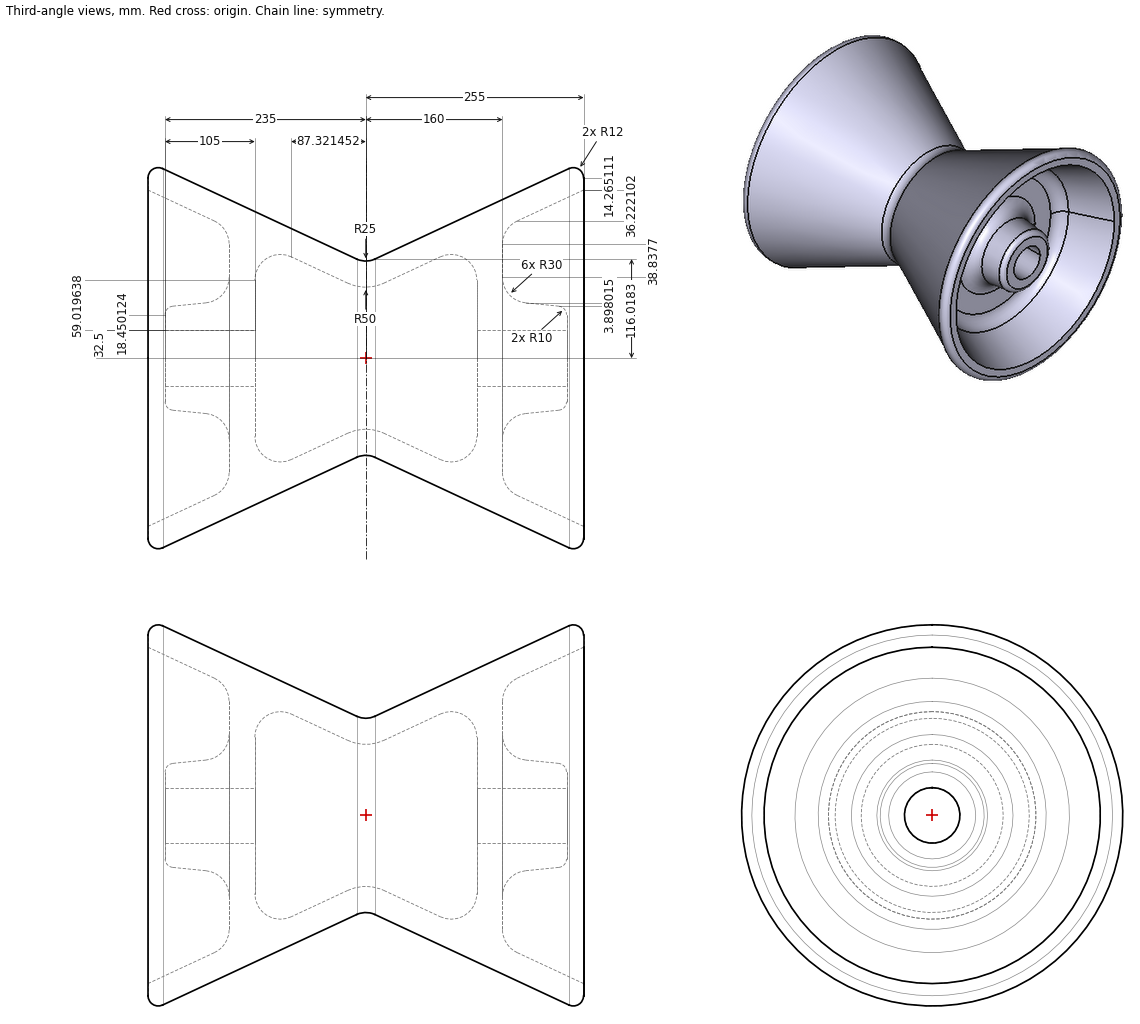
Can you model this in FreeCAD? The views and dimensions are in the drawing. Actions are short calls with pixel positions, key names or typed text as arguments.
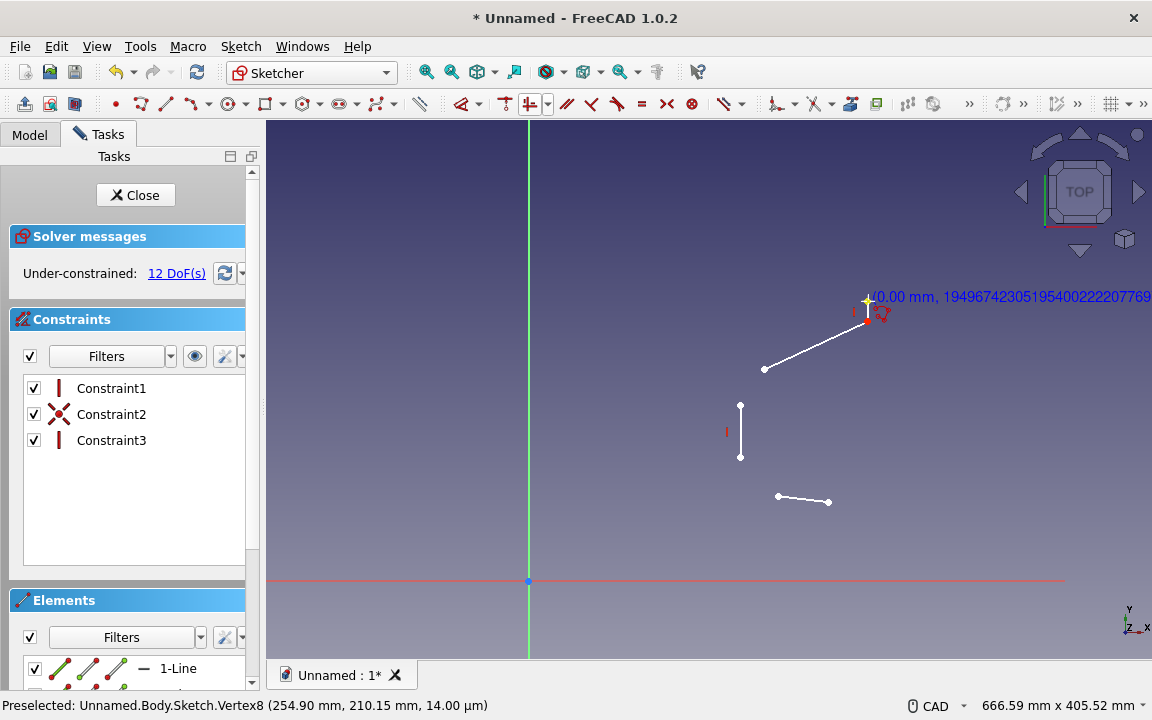
click(166, 104)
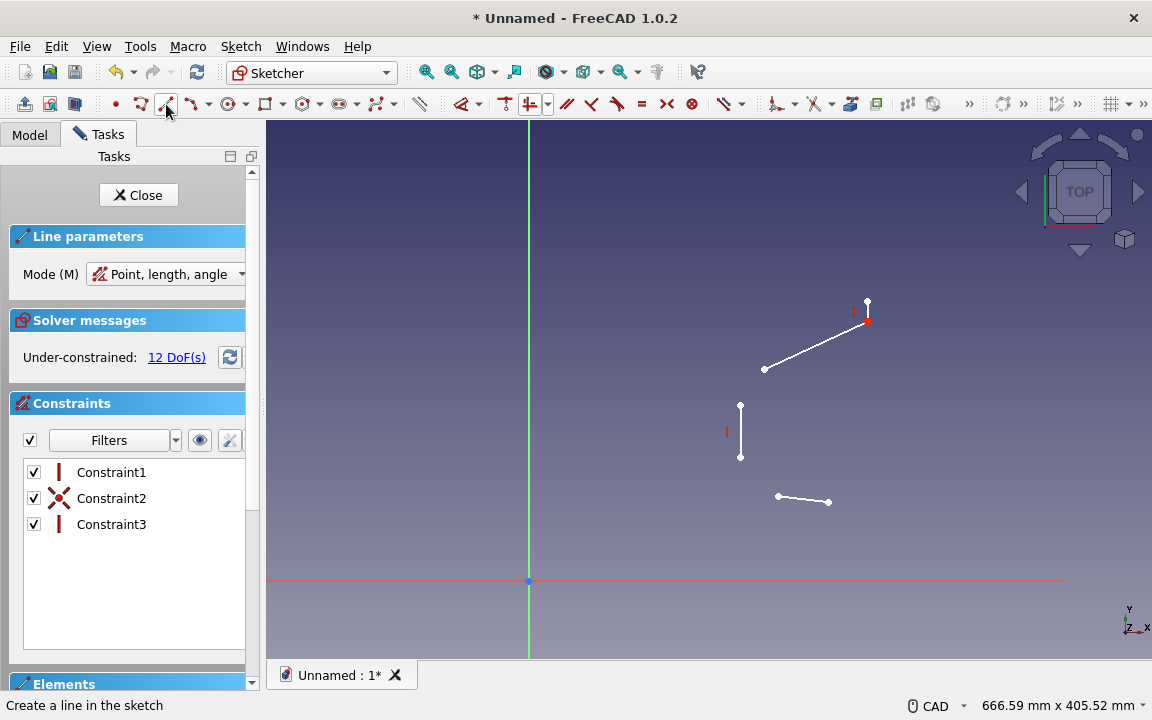
click(845, 286)
click(543, 427)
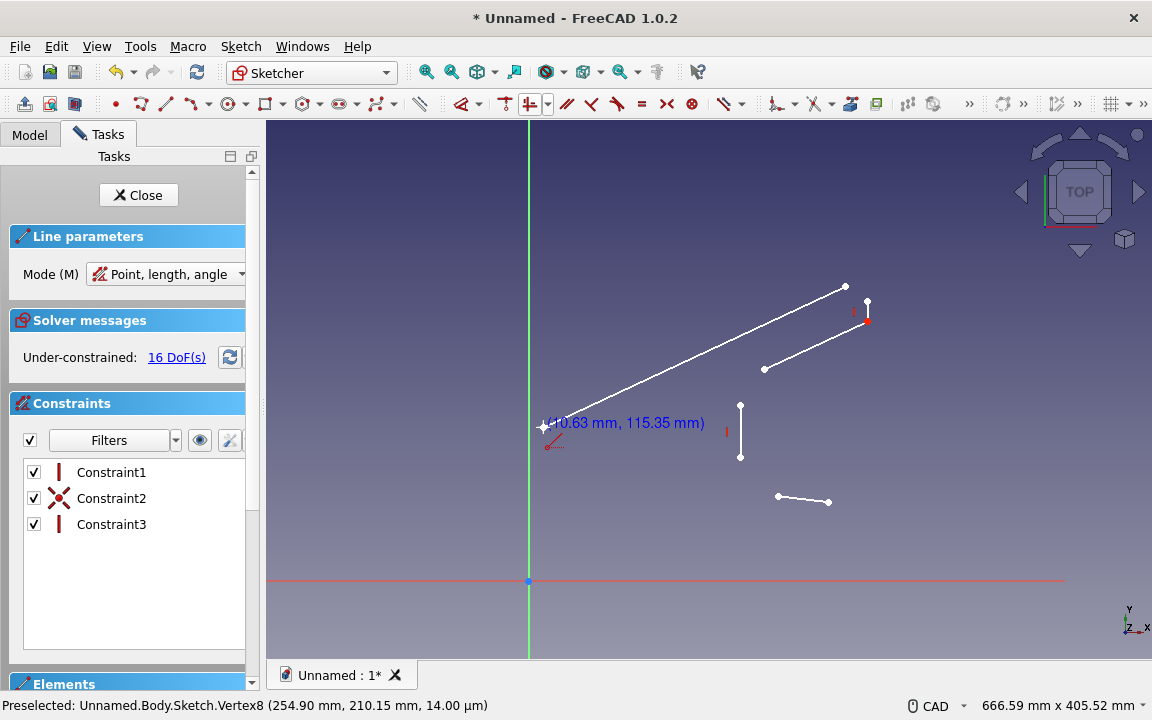
click(515, 427)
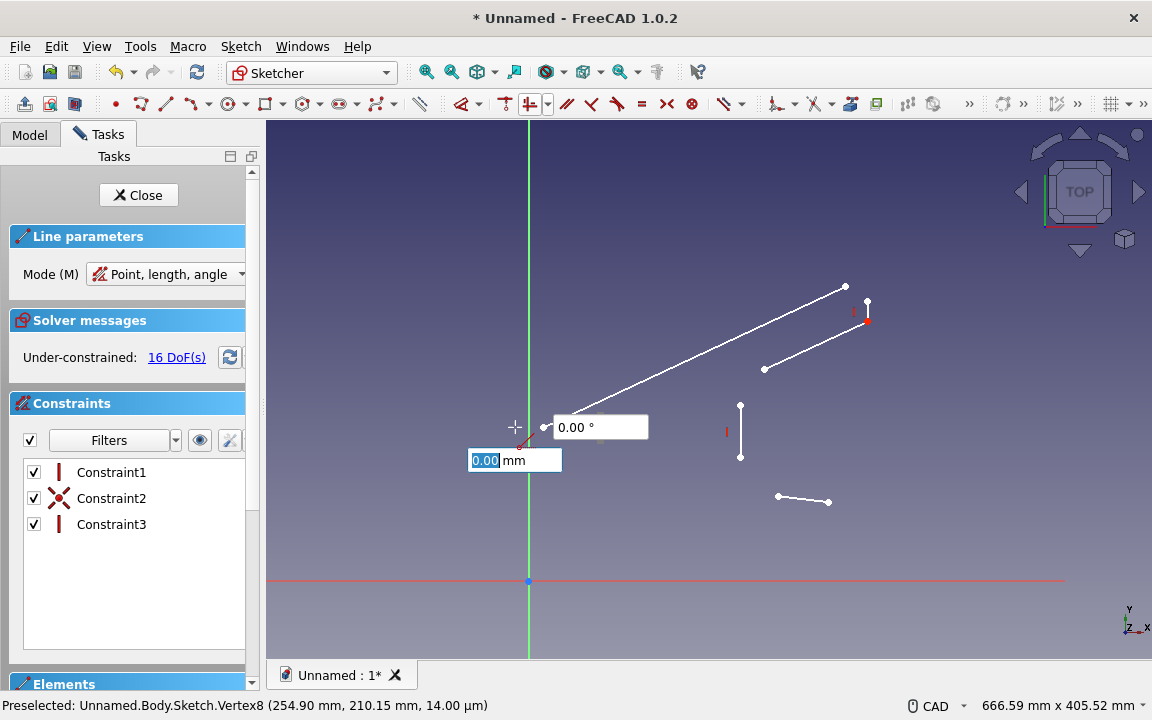
scroll(867, 300, down, 2)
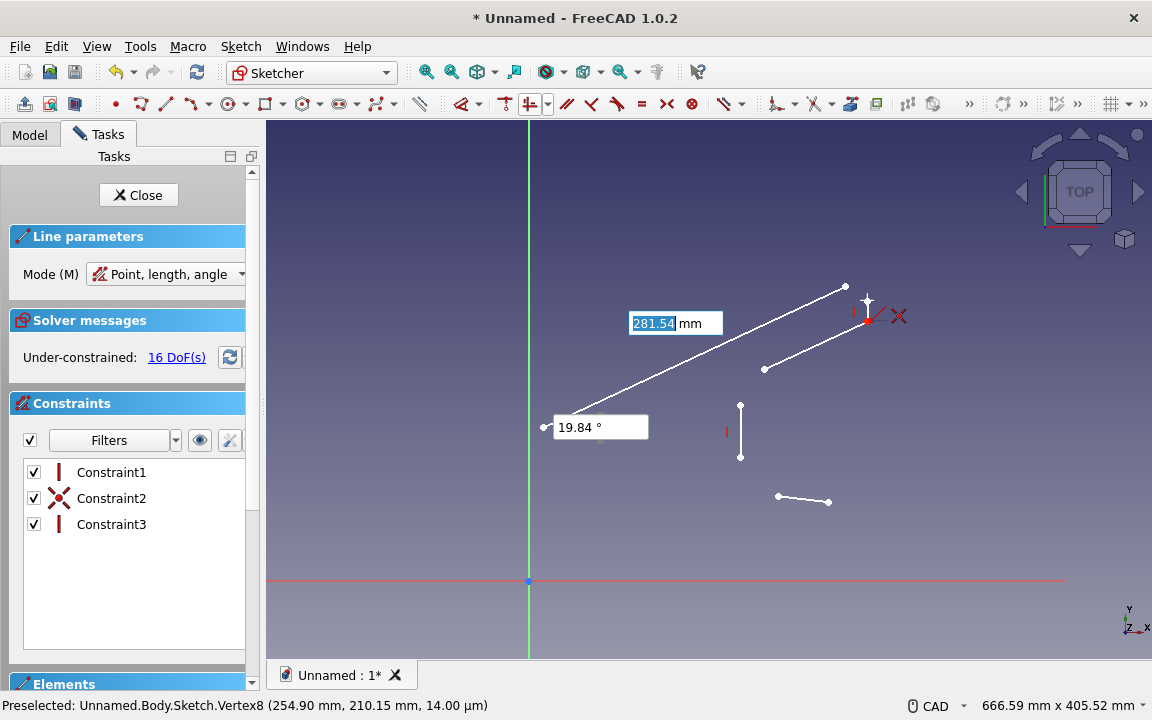
click(429, 291)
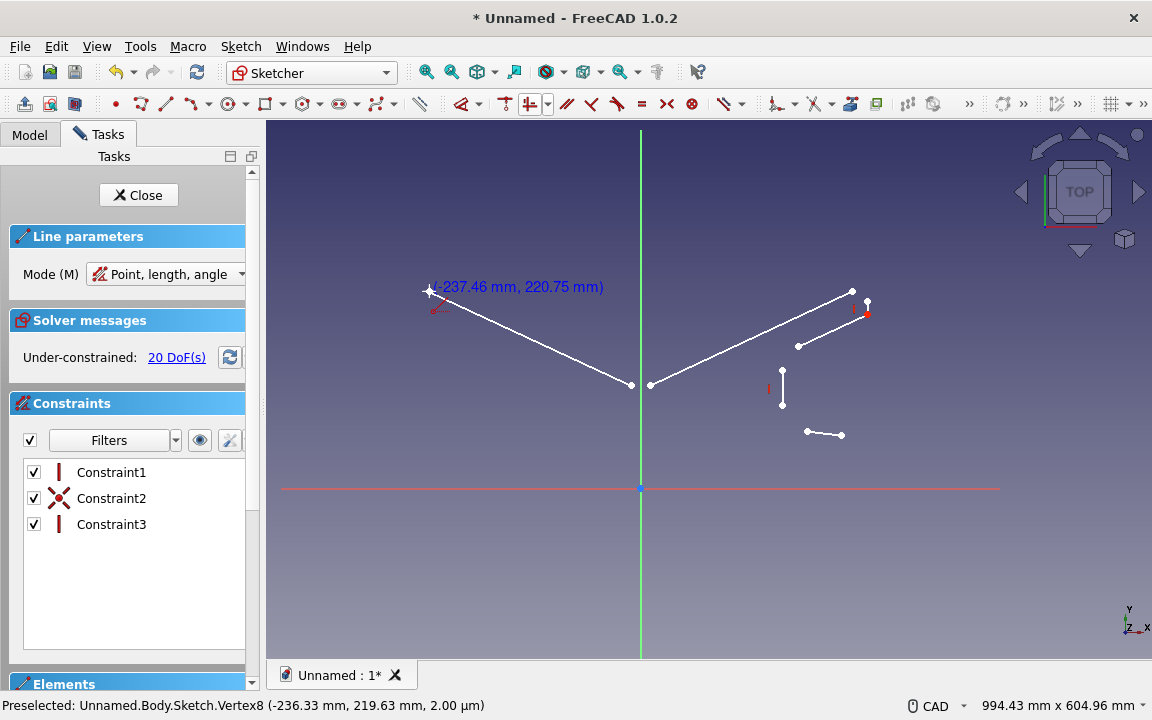
key(g)
key(m)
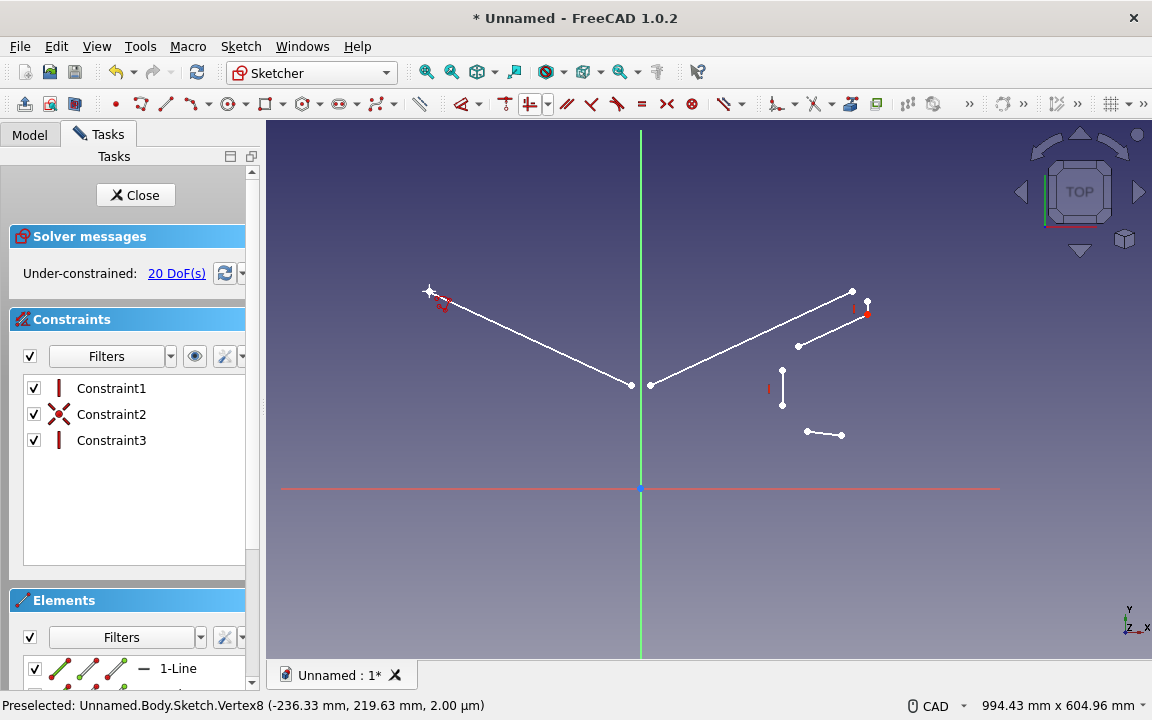
click(413, 301)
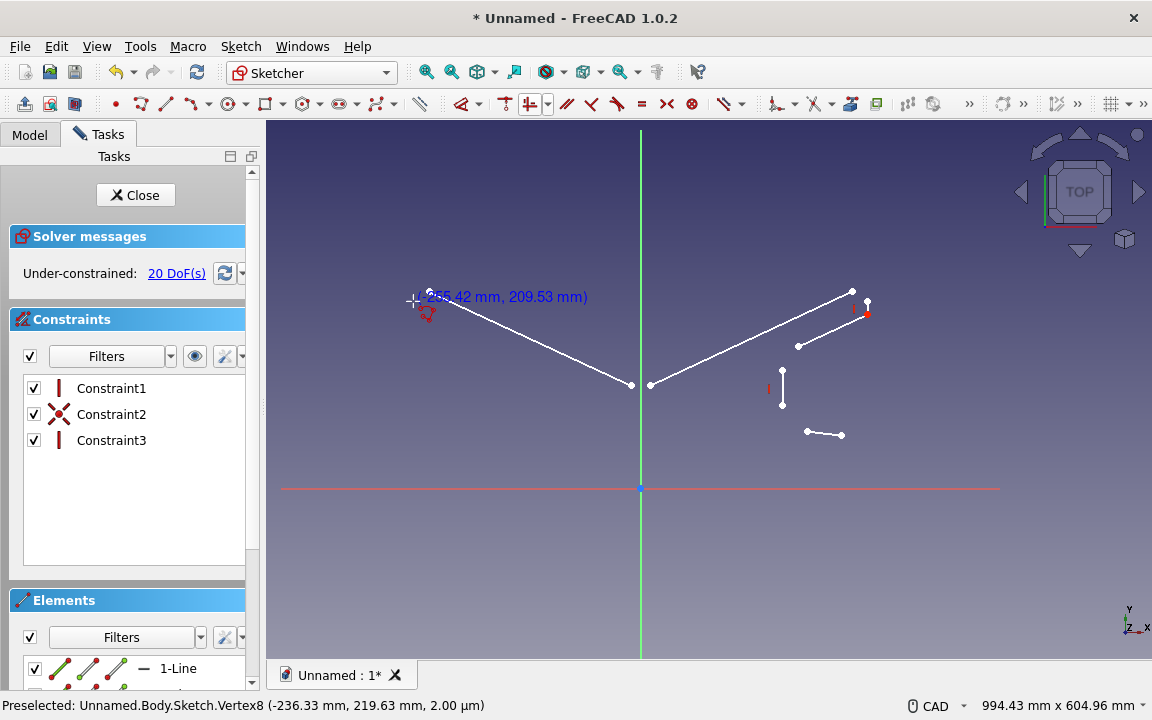
scroll(413, 313, up, 2)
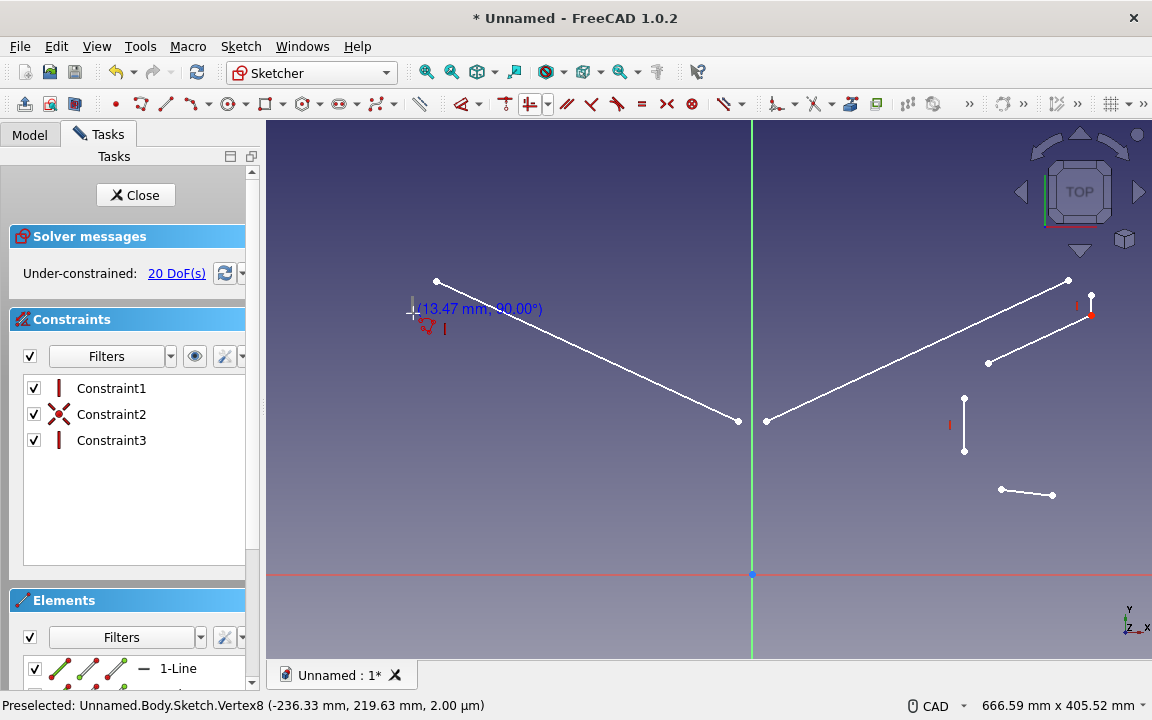
click(413, 313)
click(517, 361)
right_click(517, 361)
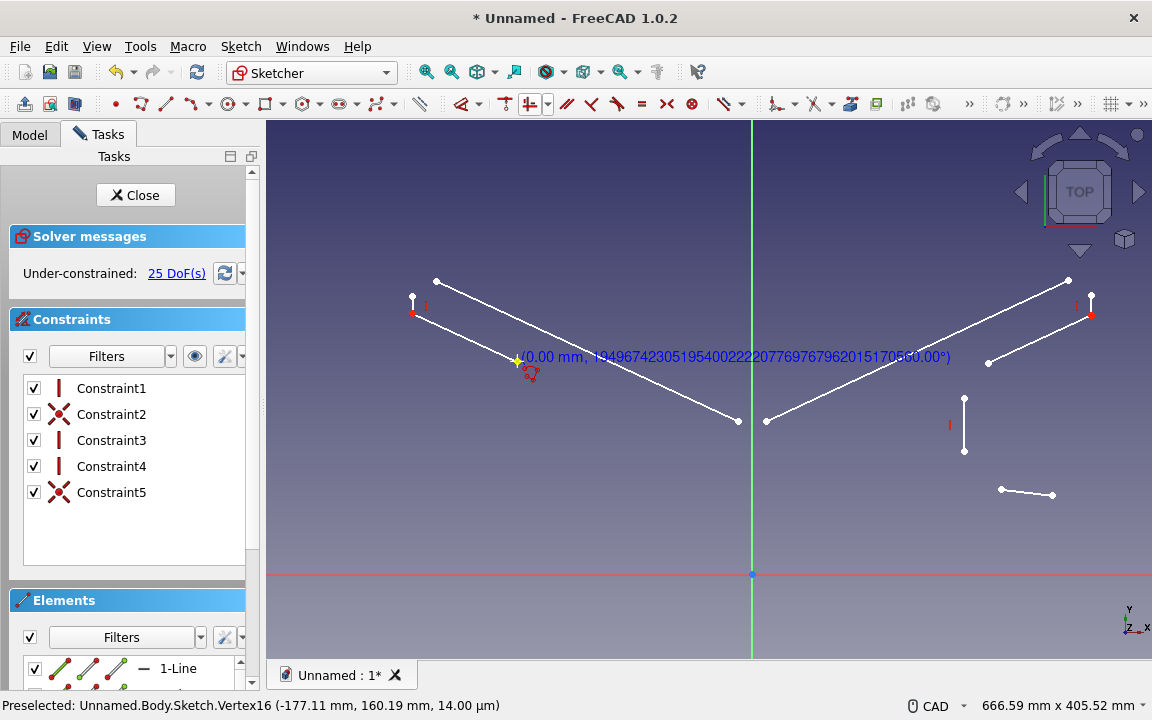
click(166, 104)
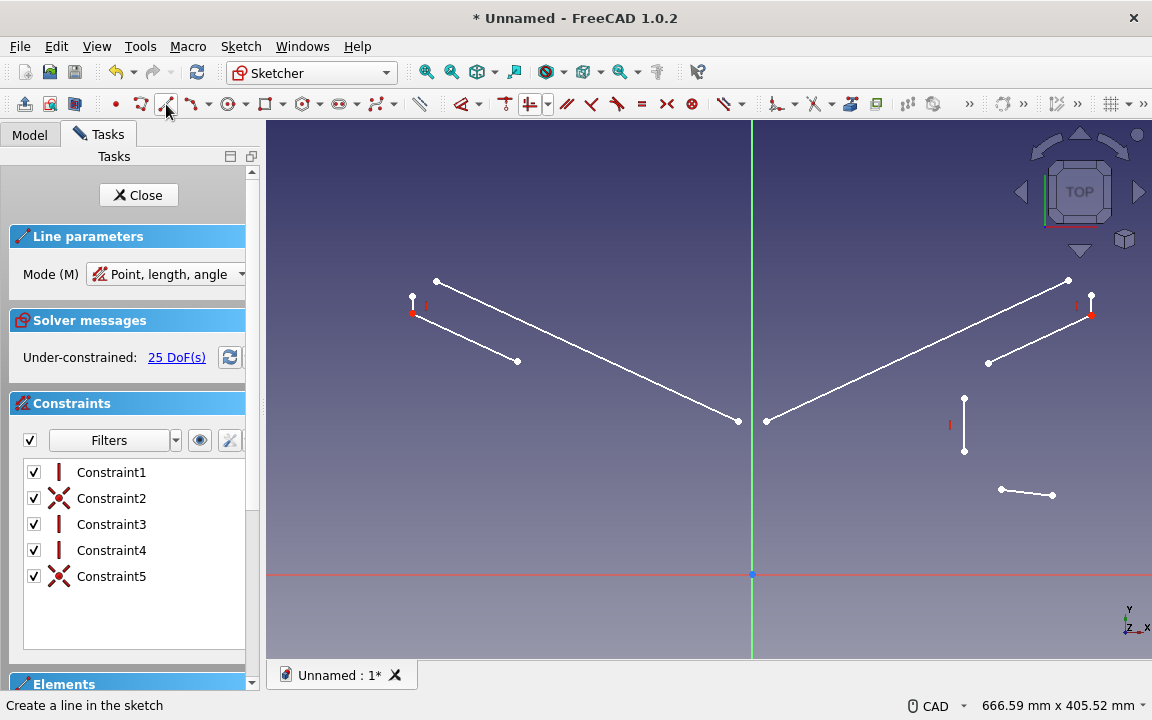
click(540, 397)
click(540, 449)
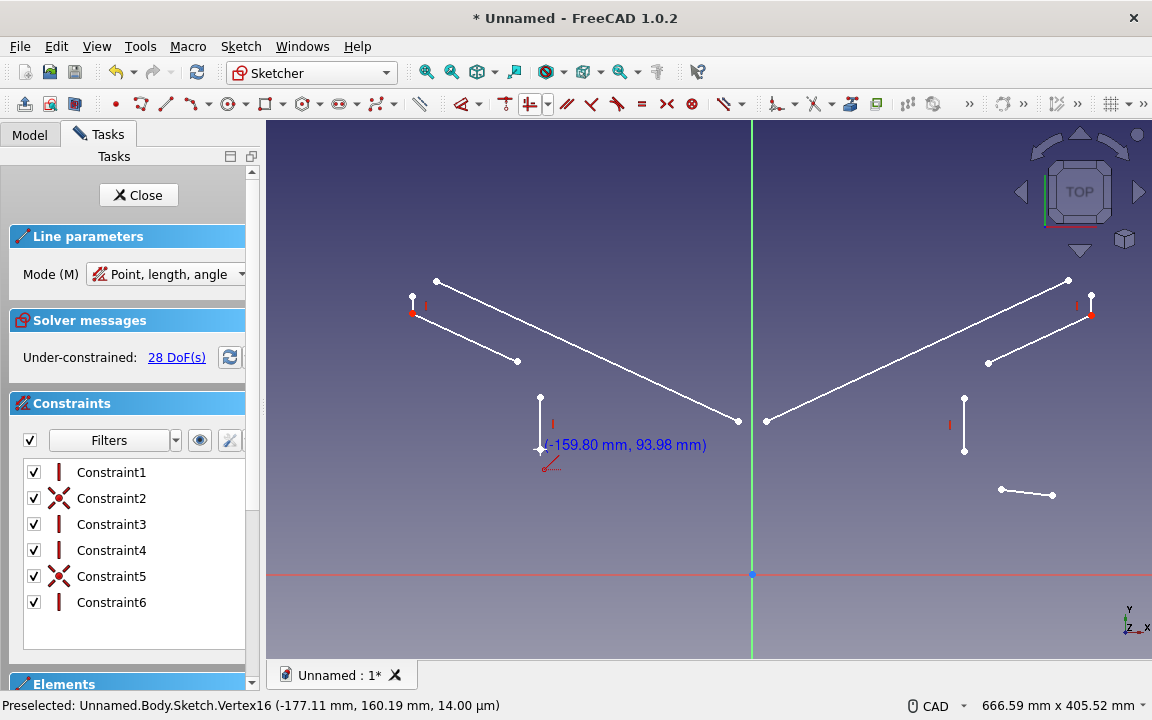
click(504, 489)
click(452, 494)